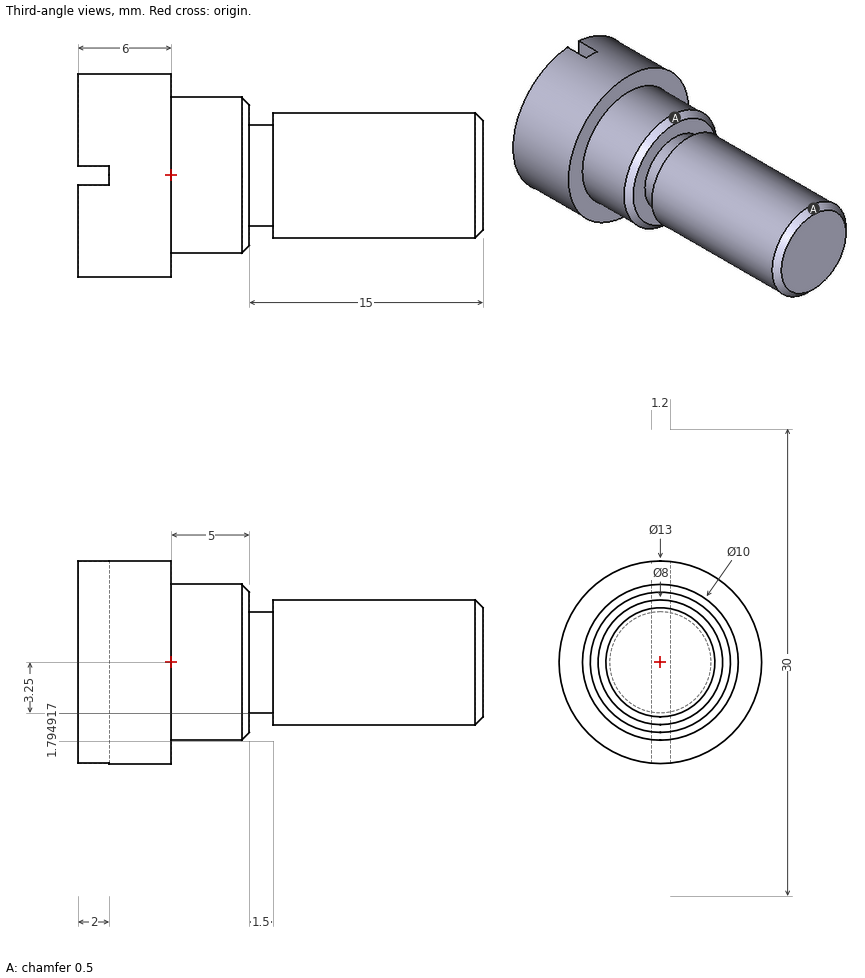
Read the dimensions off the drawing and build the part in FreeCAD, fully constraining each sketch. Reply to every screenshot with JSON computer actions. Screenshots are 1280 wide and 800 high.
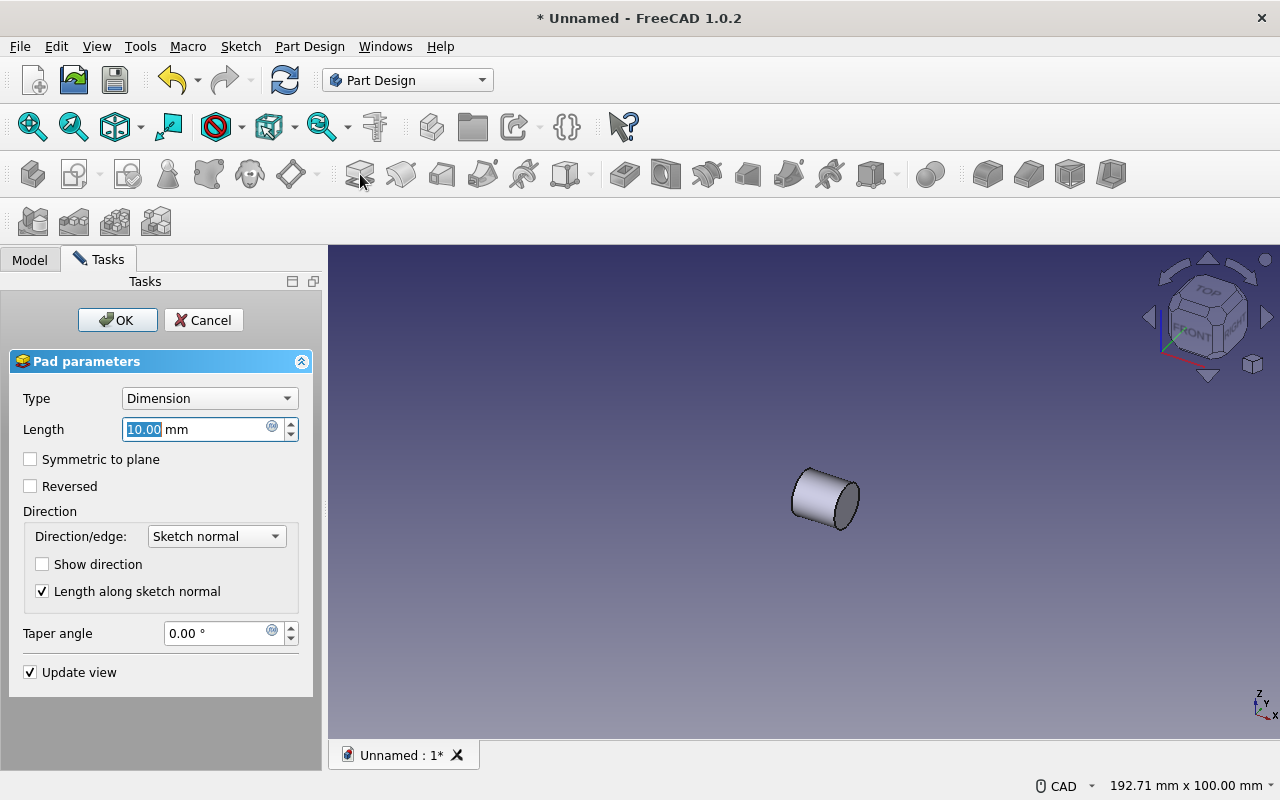
{"action": "type", "text": "5"}
{"action": "key", "text": "Tab"}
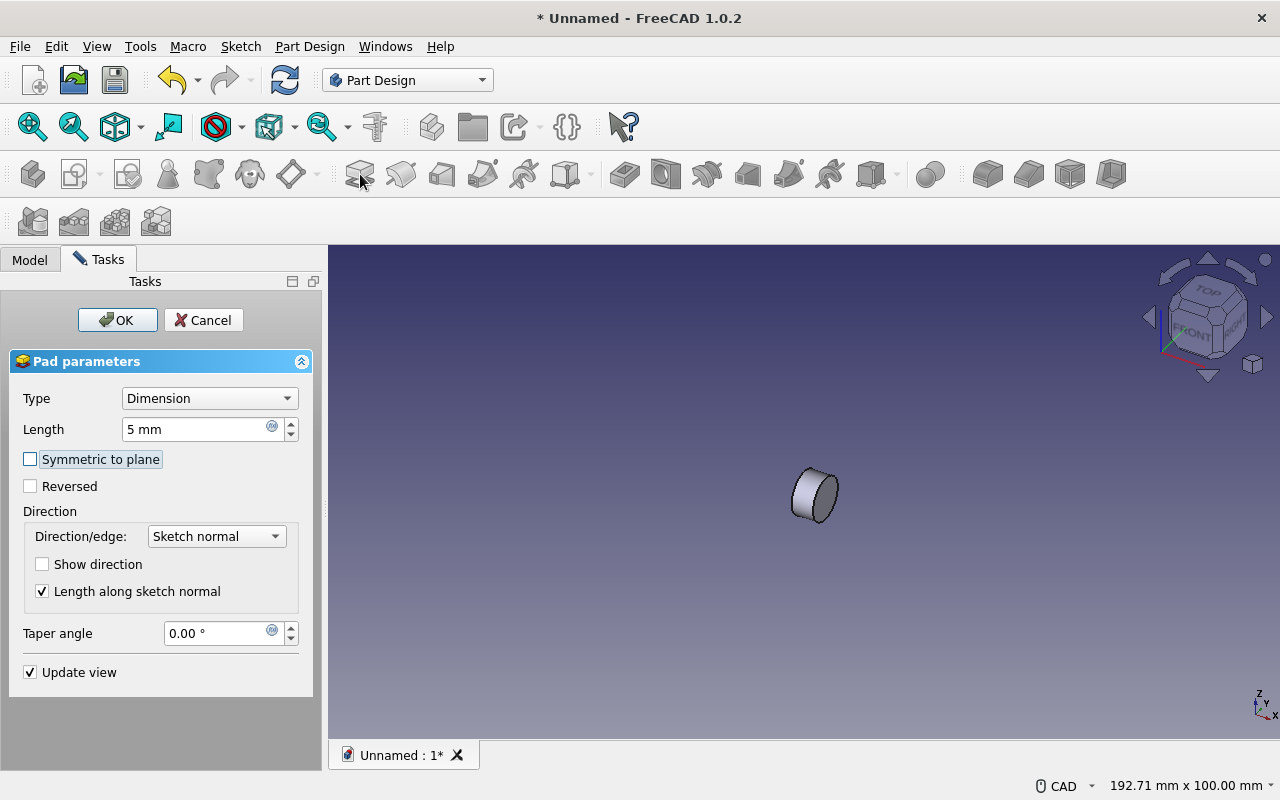
{"action": "left_click", "coordinate": [118, 320]}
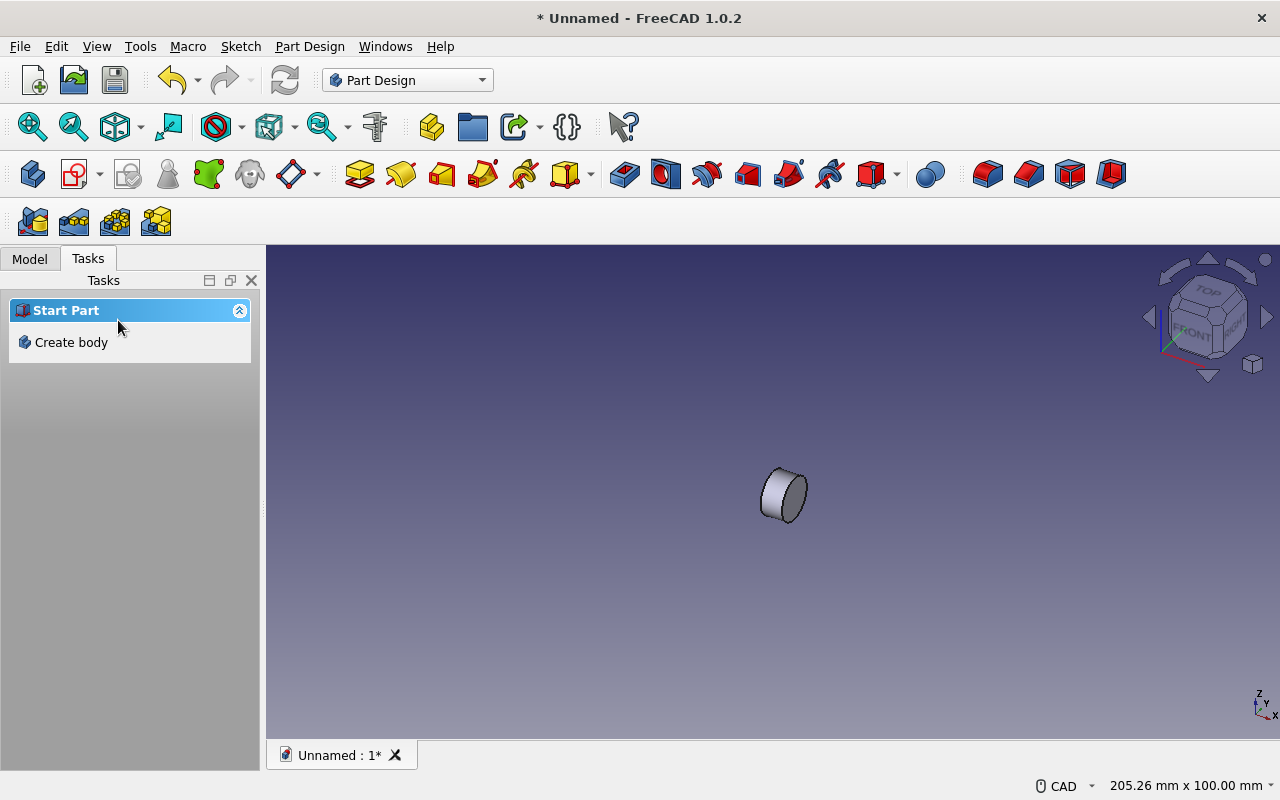
{"action": "key", "text": "v f"}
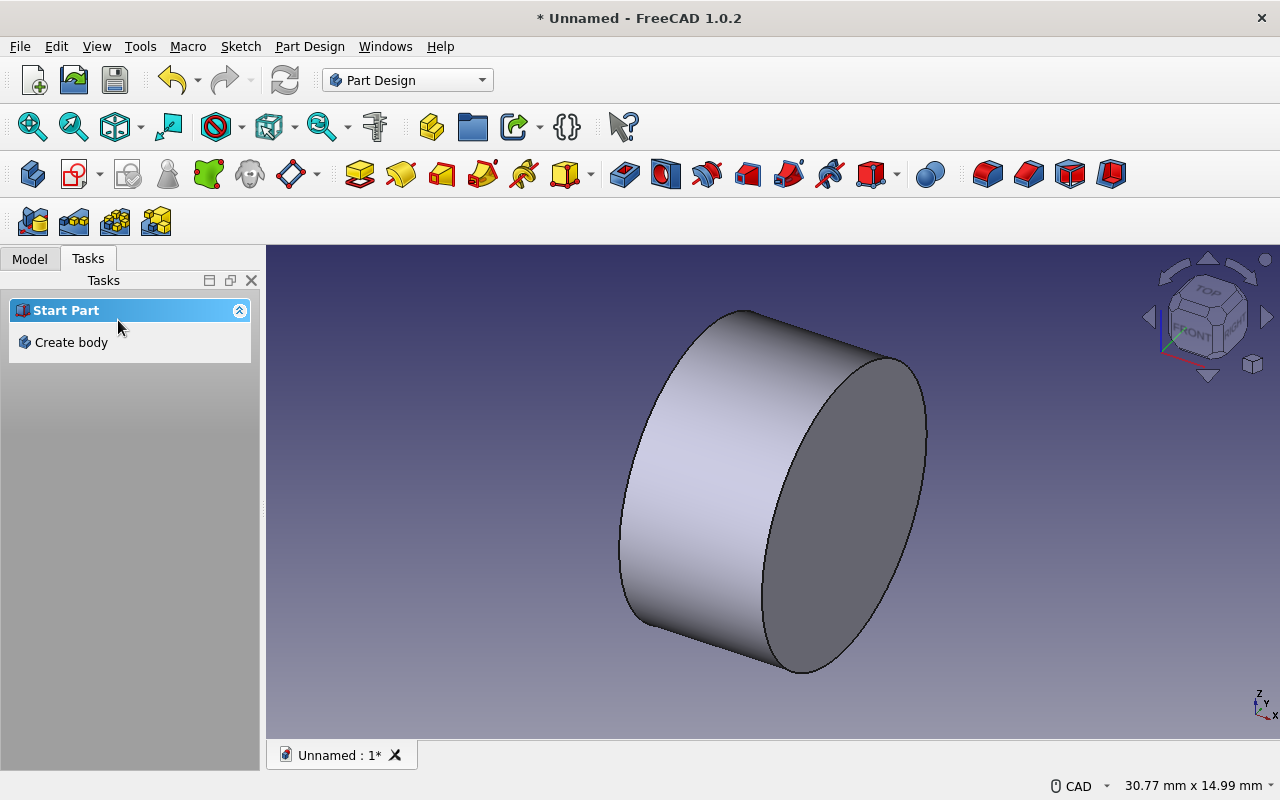
{"action": "left_click", "coordinate": [74, 174]}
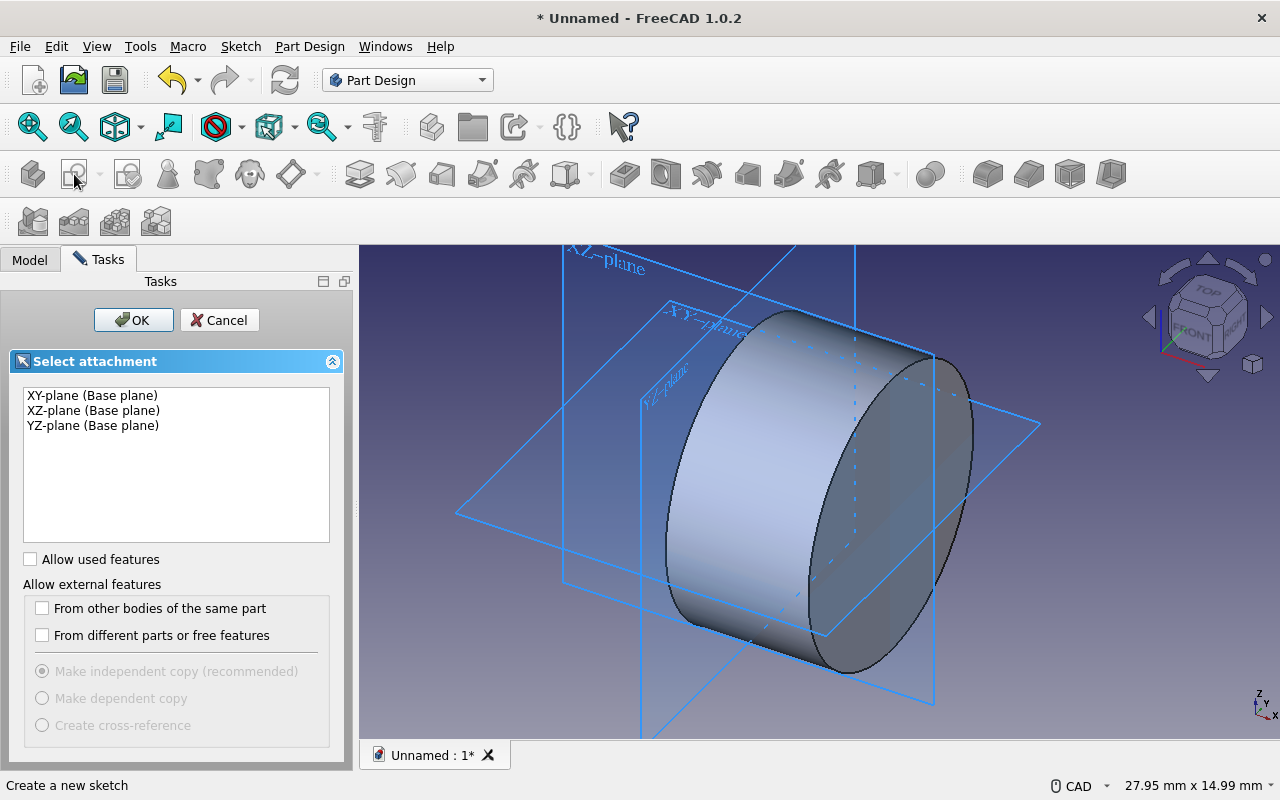
{"action": "left_click", "coordinate": [84, 426]}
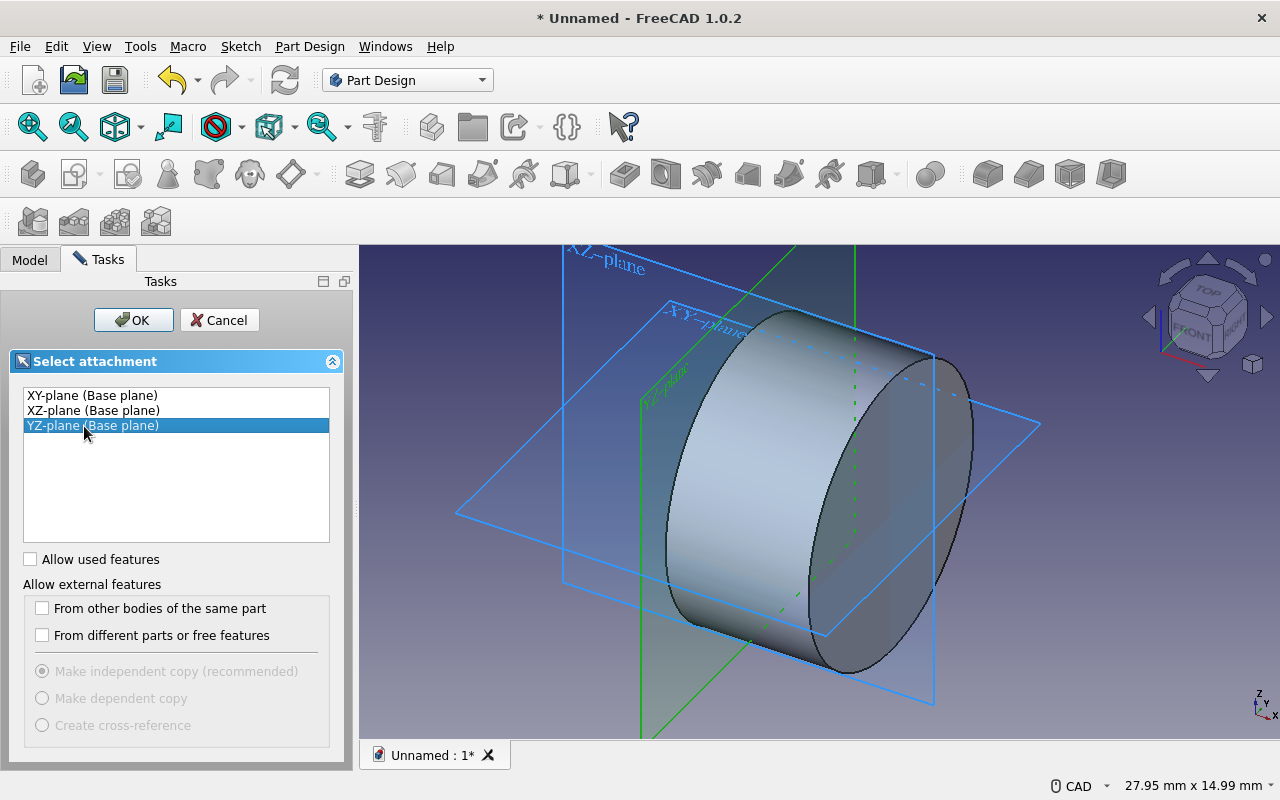
{"action": "left_click", "coordinate": [134, 320]}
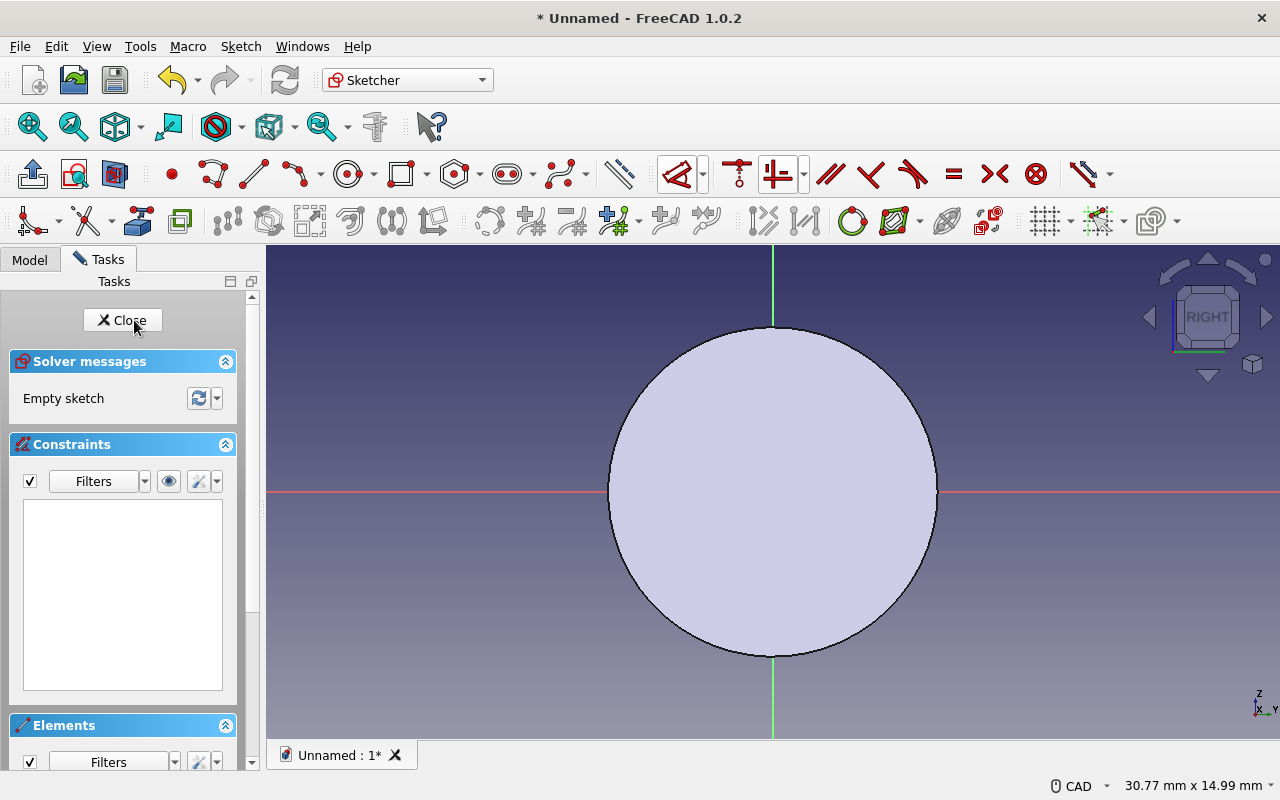
{"action": "left_click", "coordinate": [115, 174]}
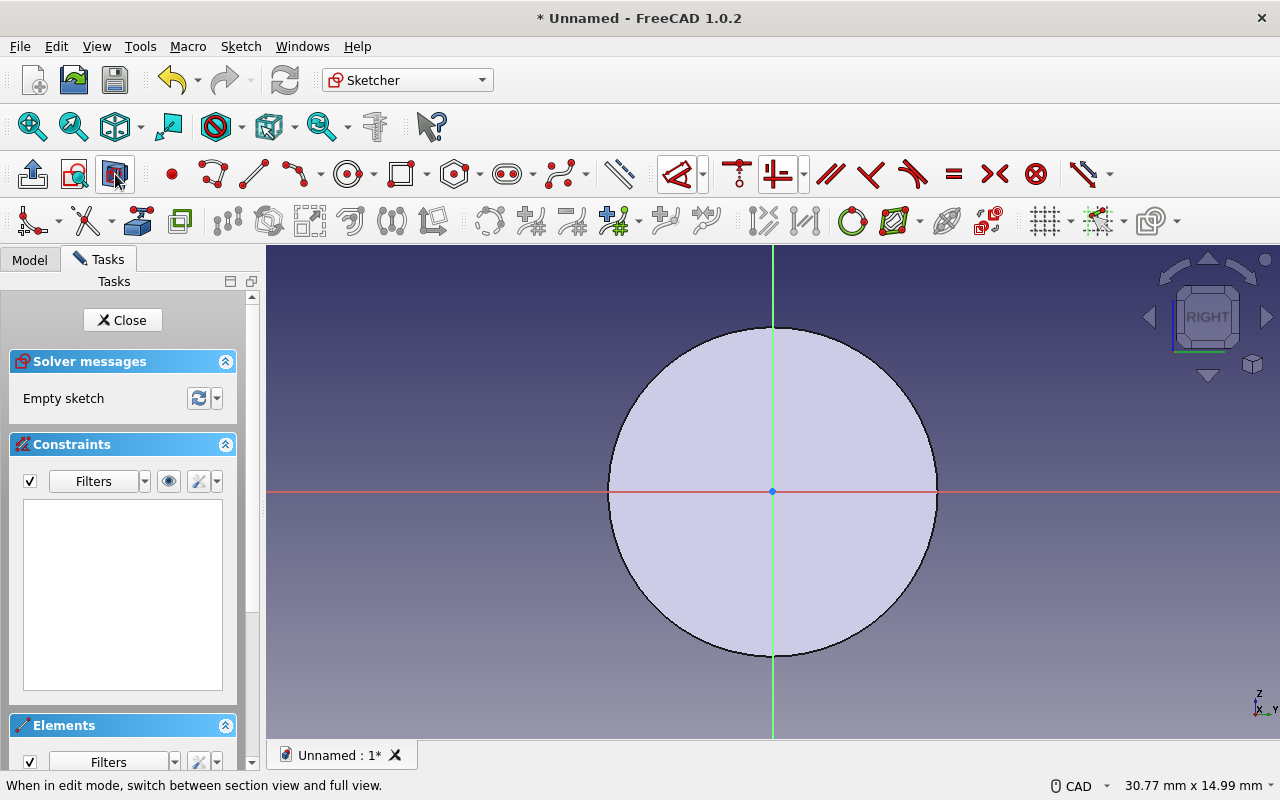
{"action": "scroll", "coordinate": [565, 492], "scroll_direction": "down", "scroll_amount": 2}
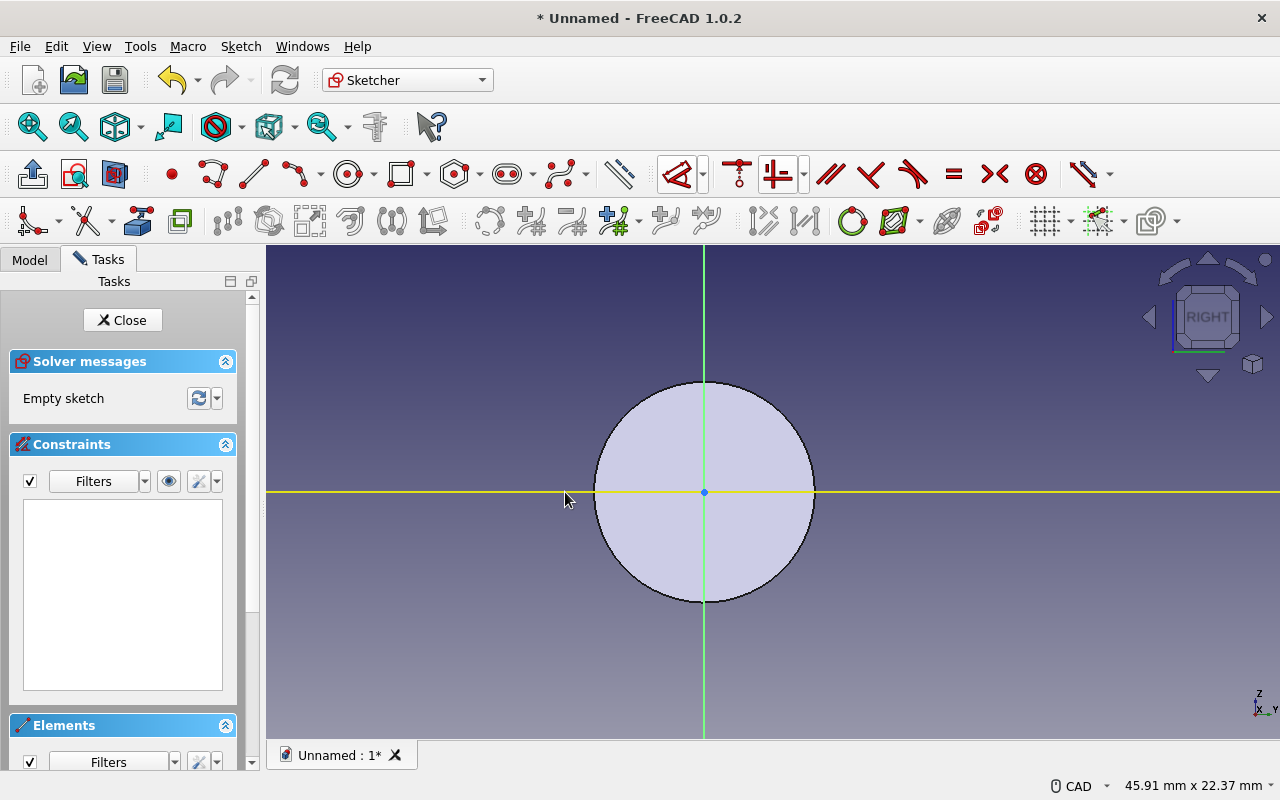
{"action": "key", "text": "g c"}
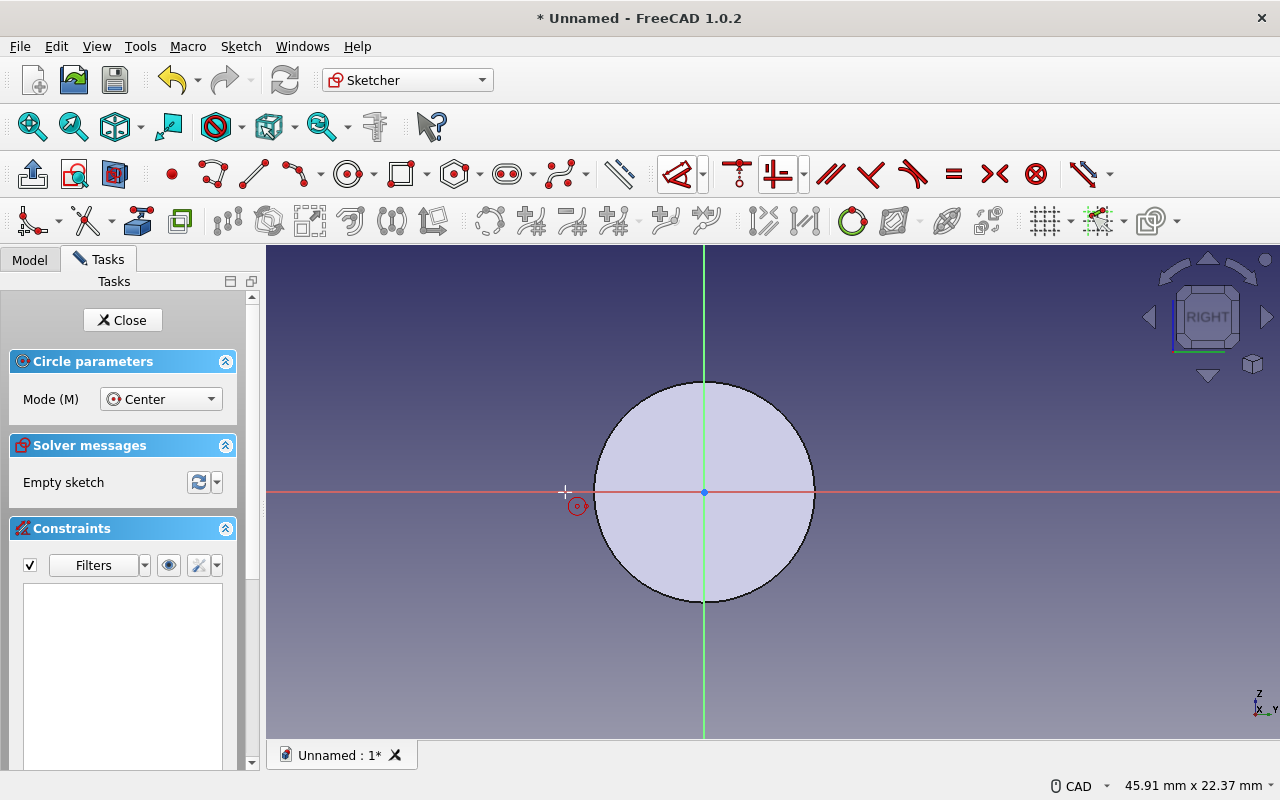
{"action": "left_click", "coordinate": [704, 492]}
{"action": "mouse_move", "coordinate": [806, 391]}